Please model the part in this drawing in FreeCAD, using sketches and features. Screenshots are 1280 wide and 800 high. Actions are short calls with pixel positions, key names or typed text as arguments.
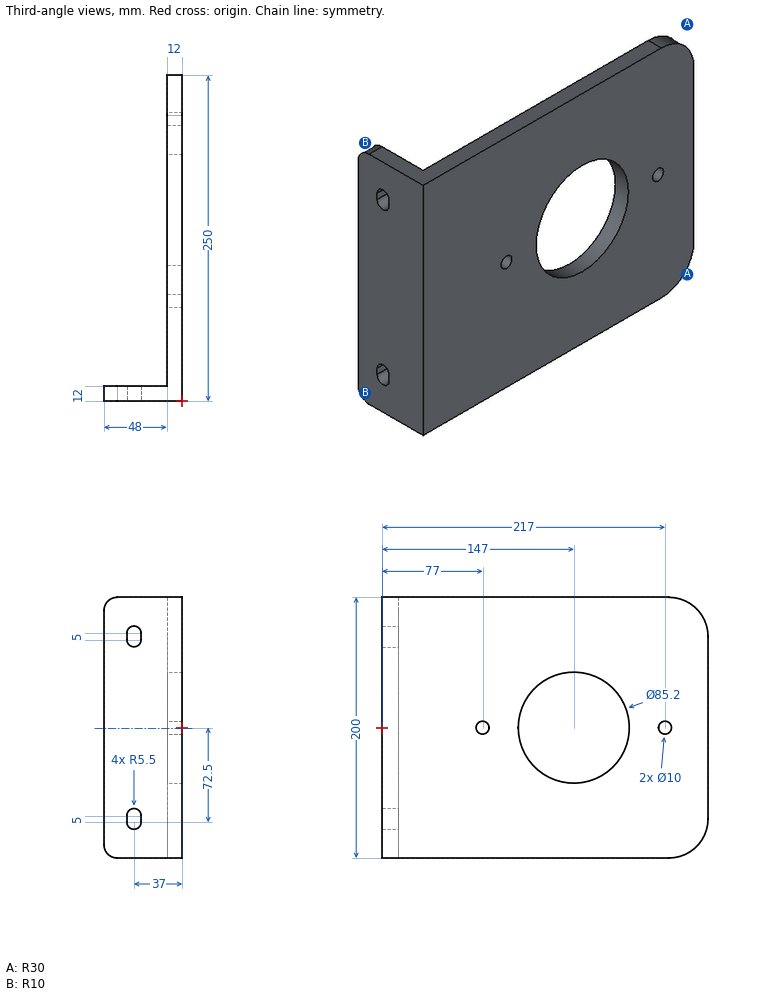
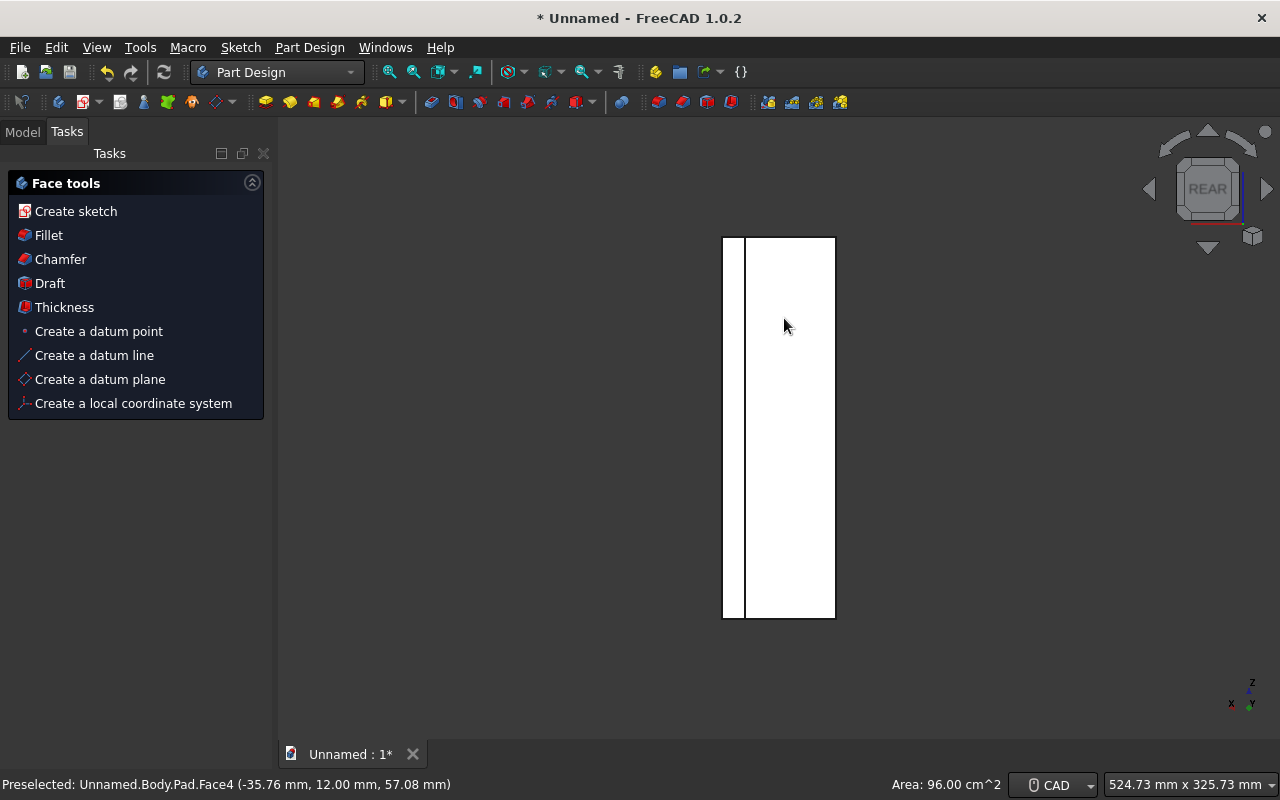
click(84, 102)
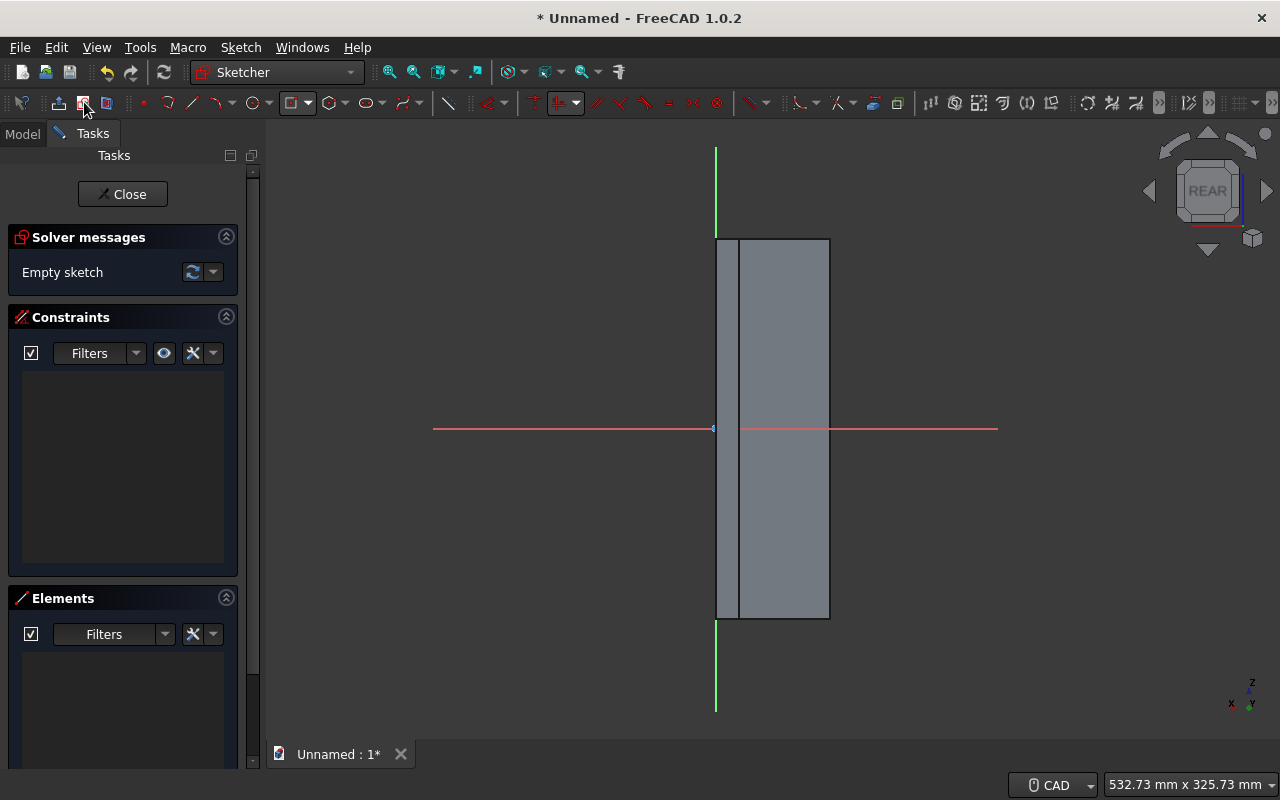
key(q)
key(s)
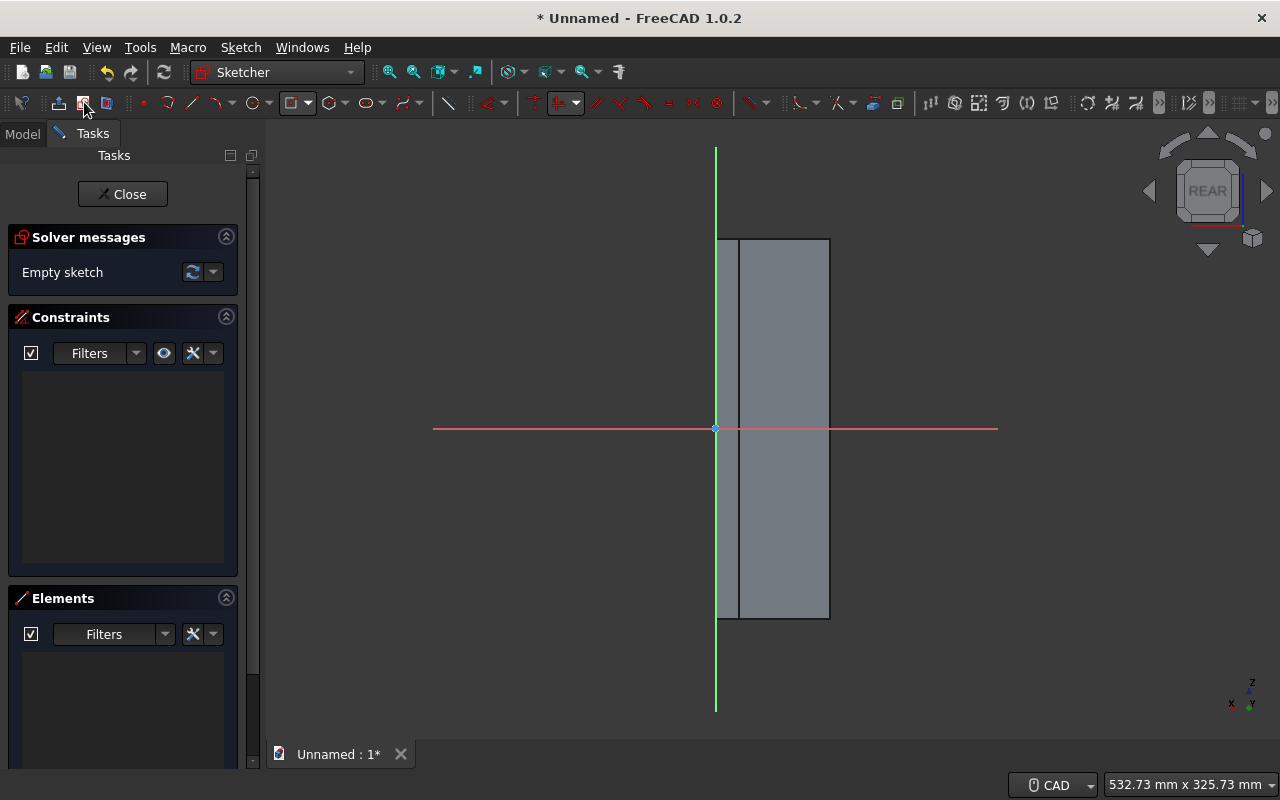
key(g)
key(s)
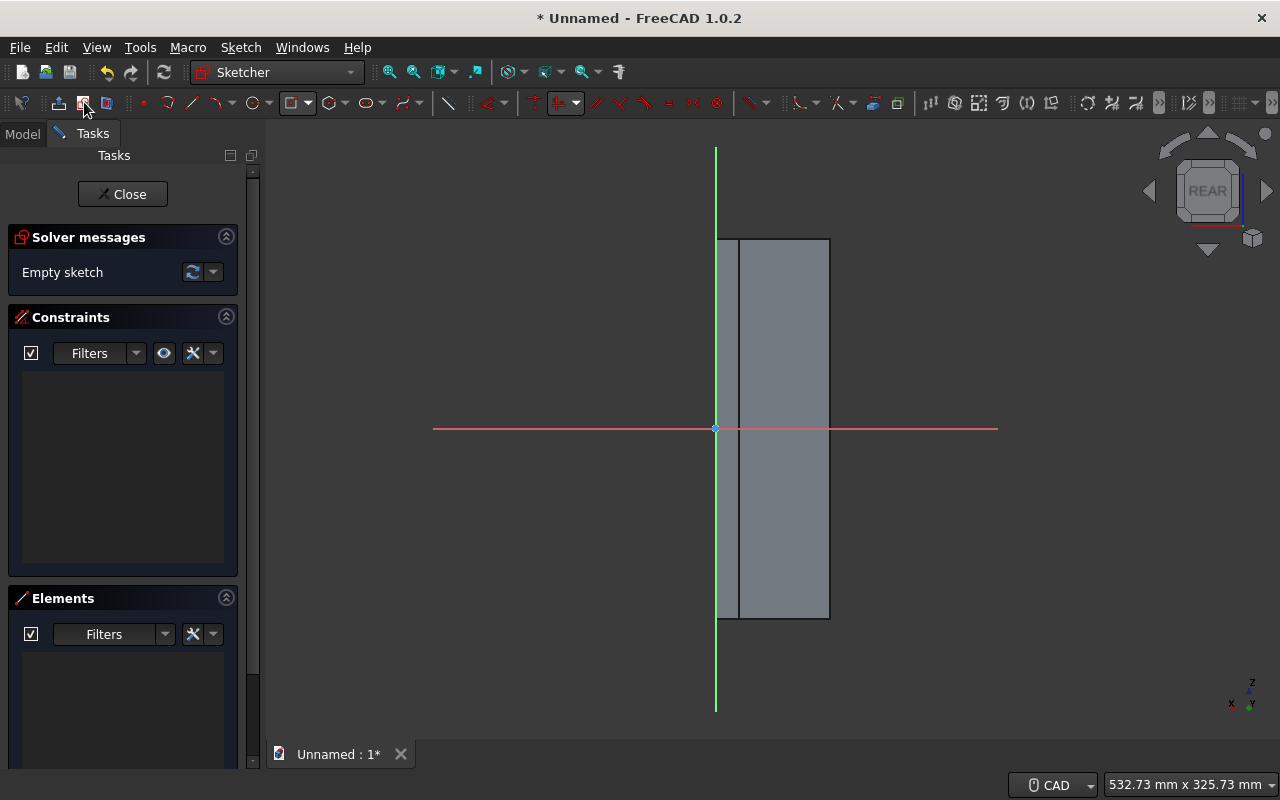
scroll(786, 567, up, 4)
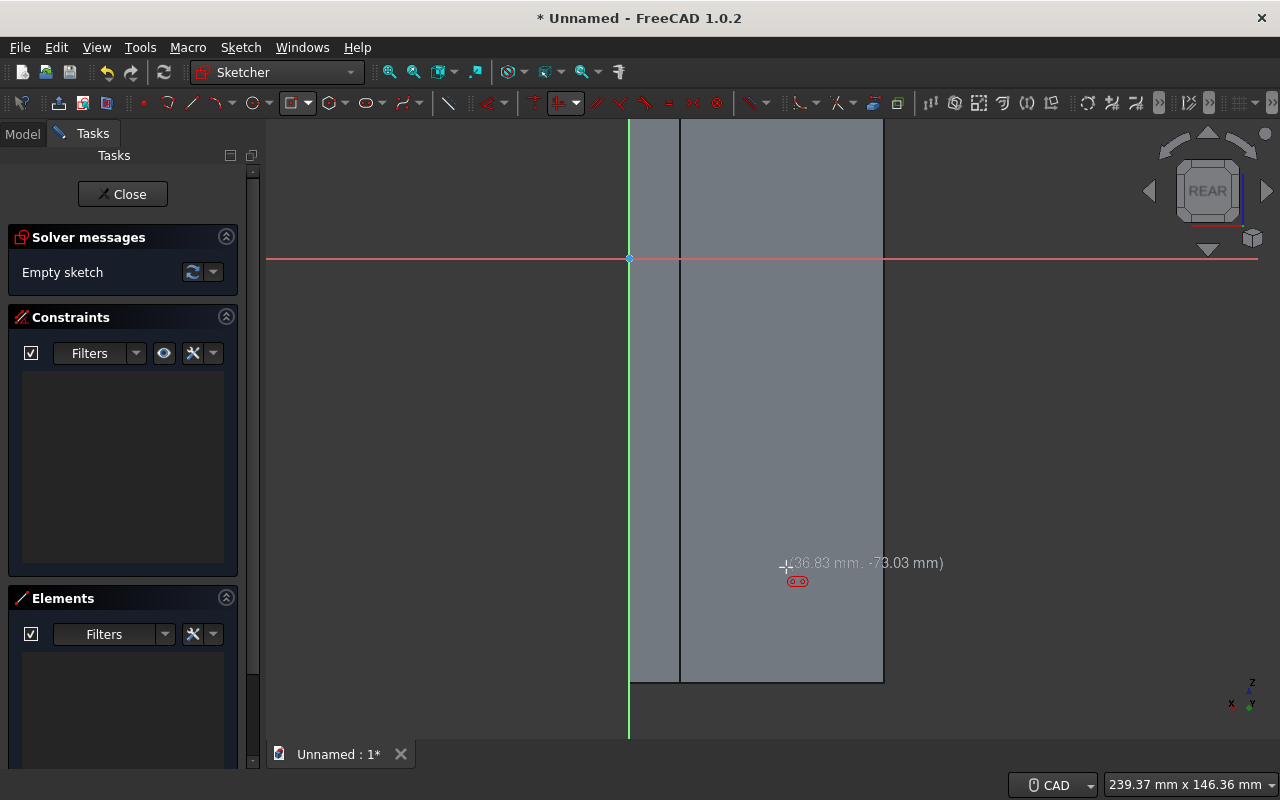
click(786, 566)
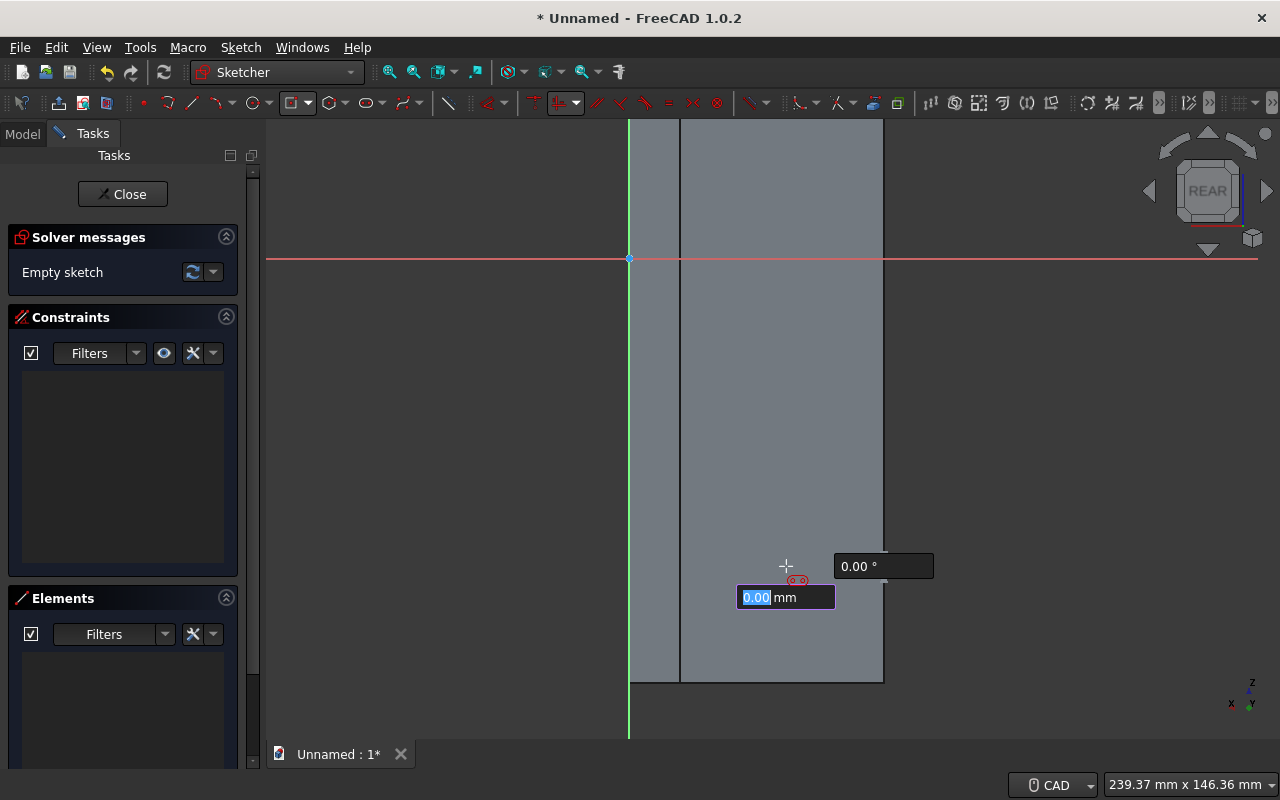
click(786, 545)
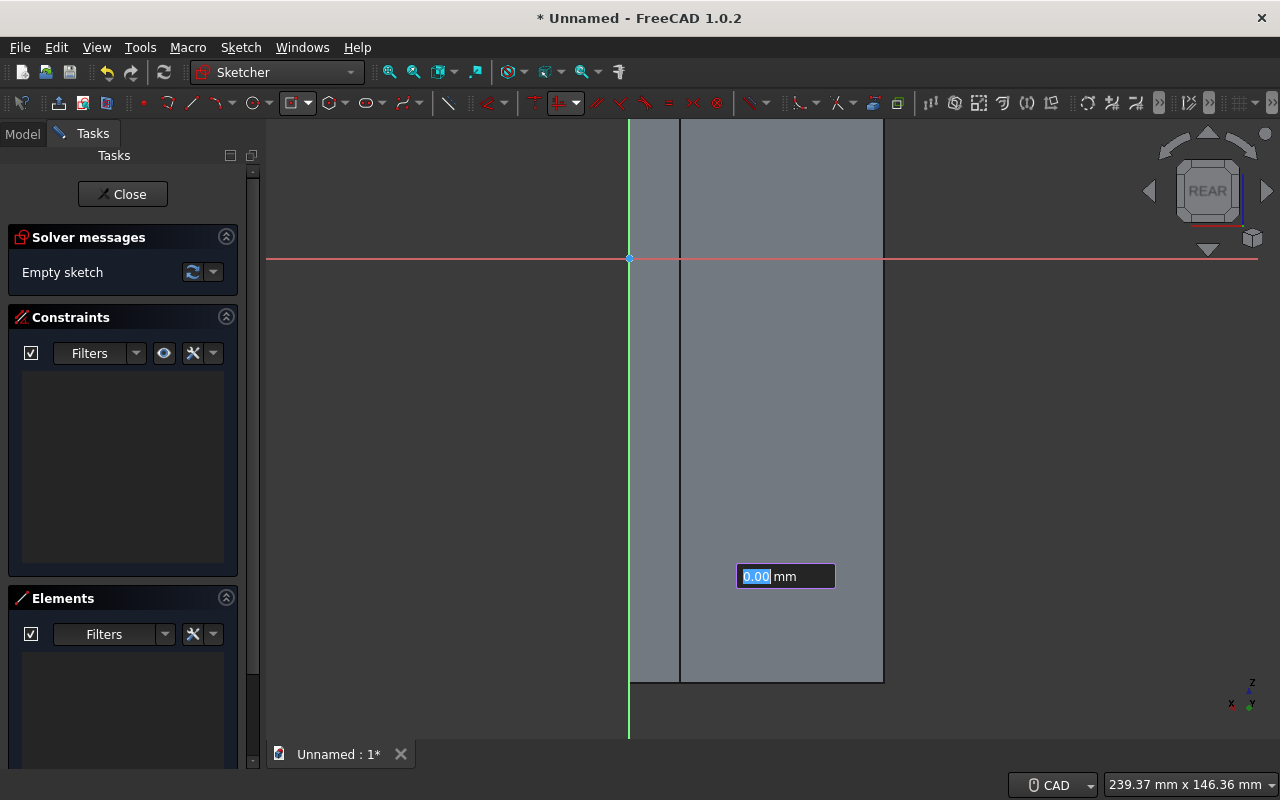
click(809, 556)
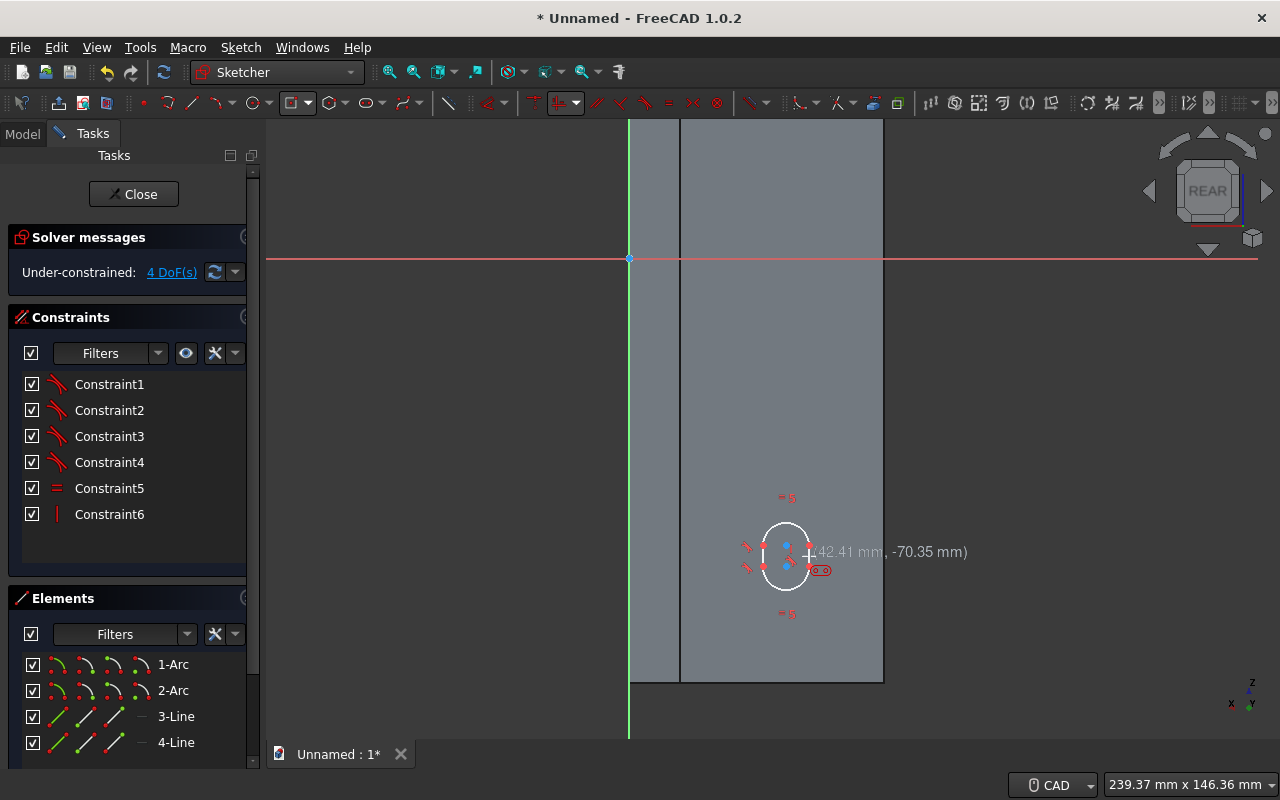
scroll(686, 636, down, 3)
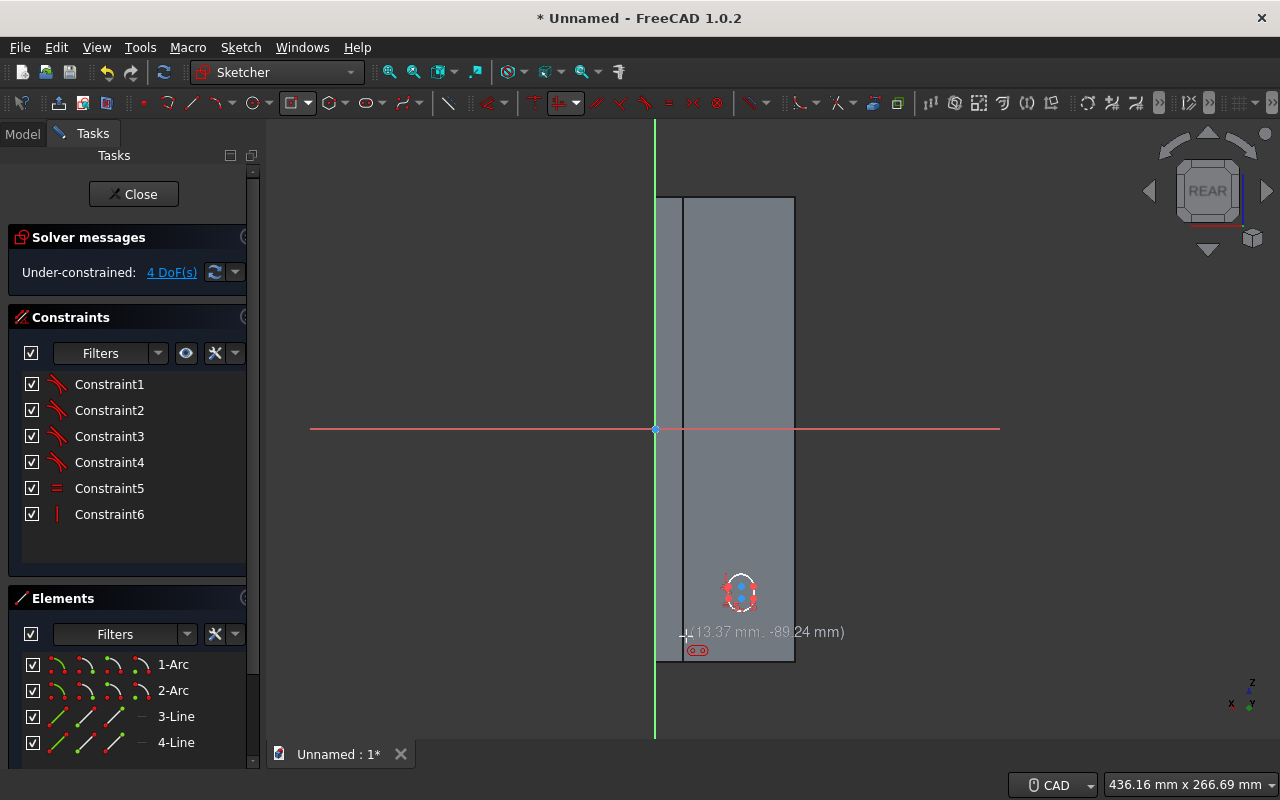
scroll(741, 273, up, 3)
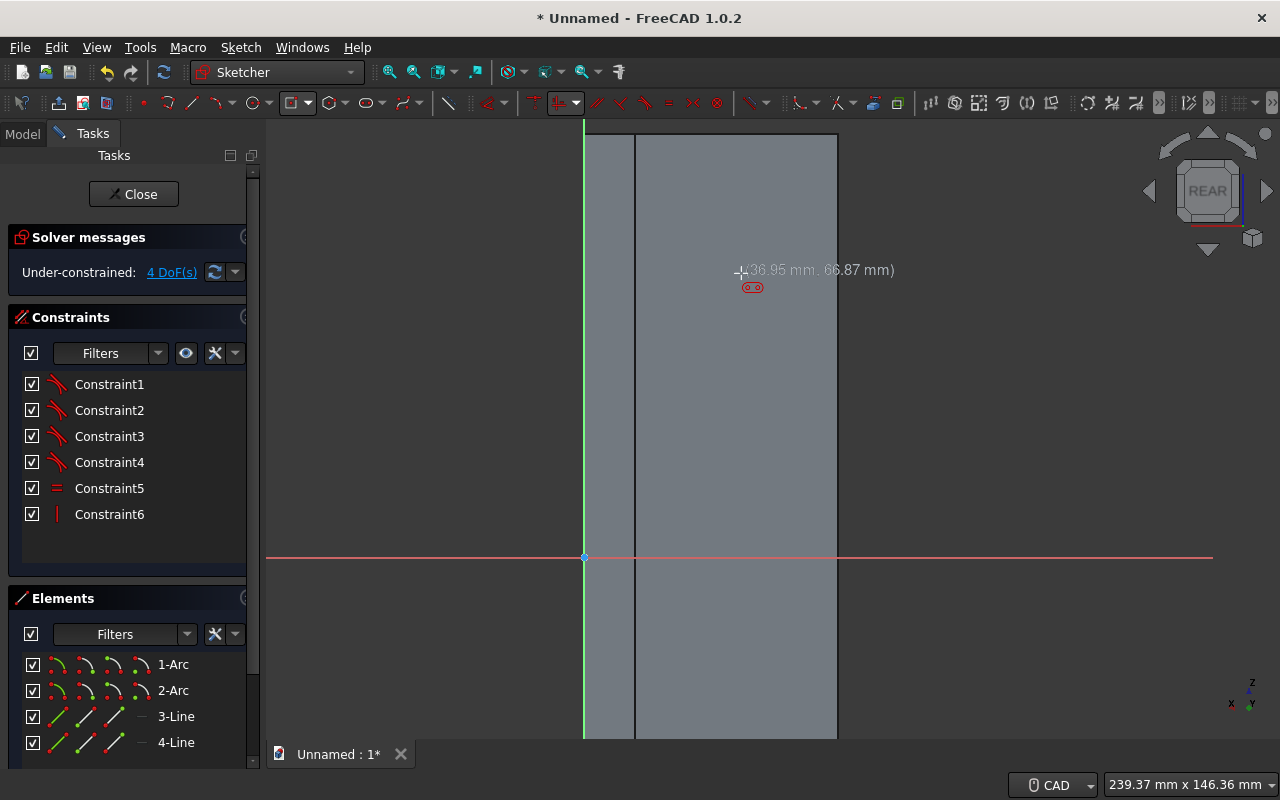
click(741, 272)